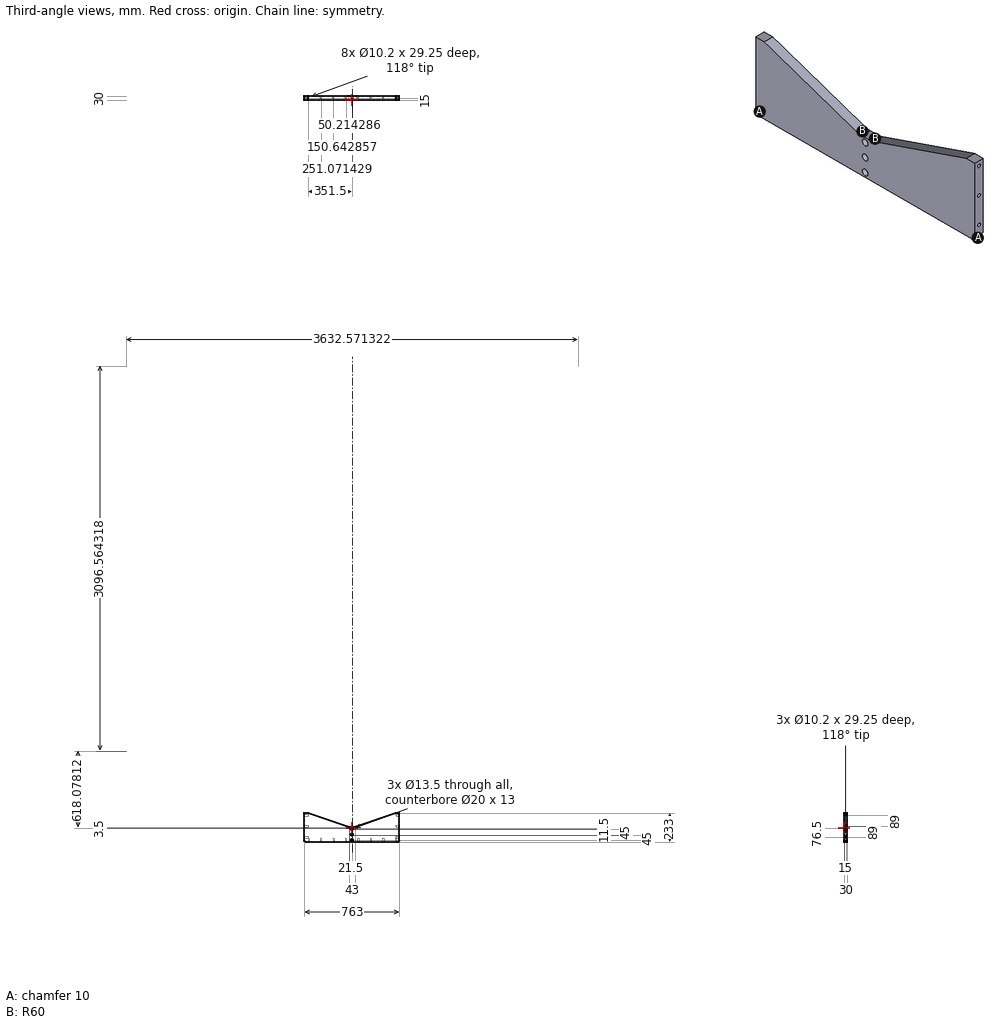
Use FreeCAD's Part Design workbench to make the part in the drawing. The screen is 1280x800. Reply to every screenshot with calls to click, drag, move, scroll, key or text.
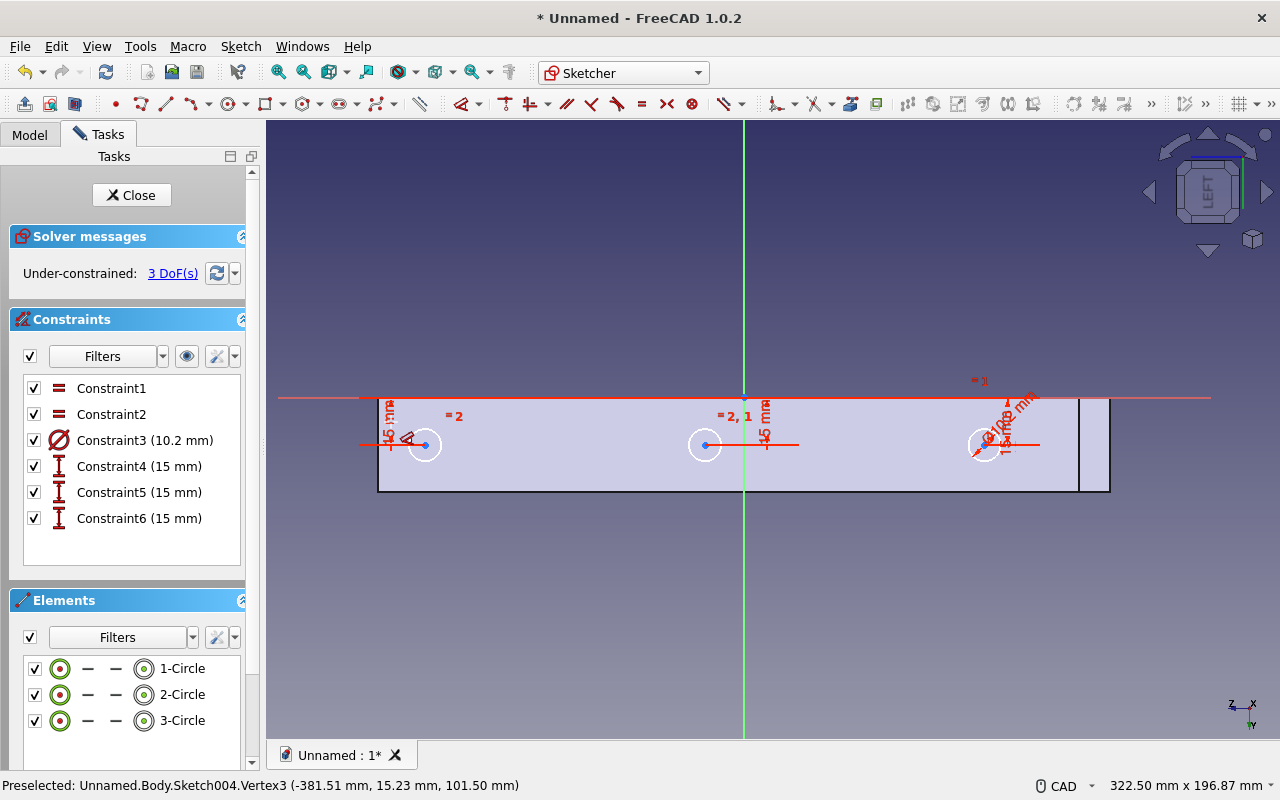
click(985, 445)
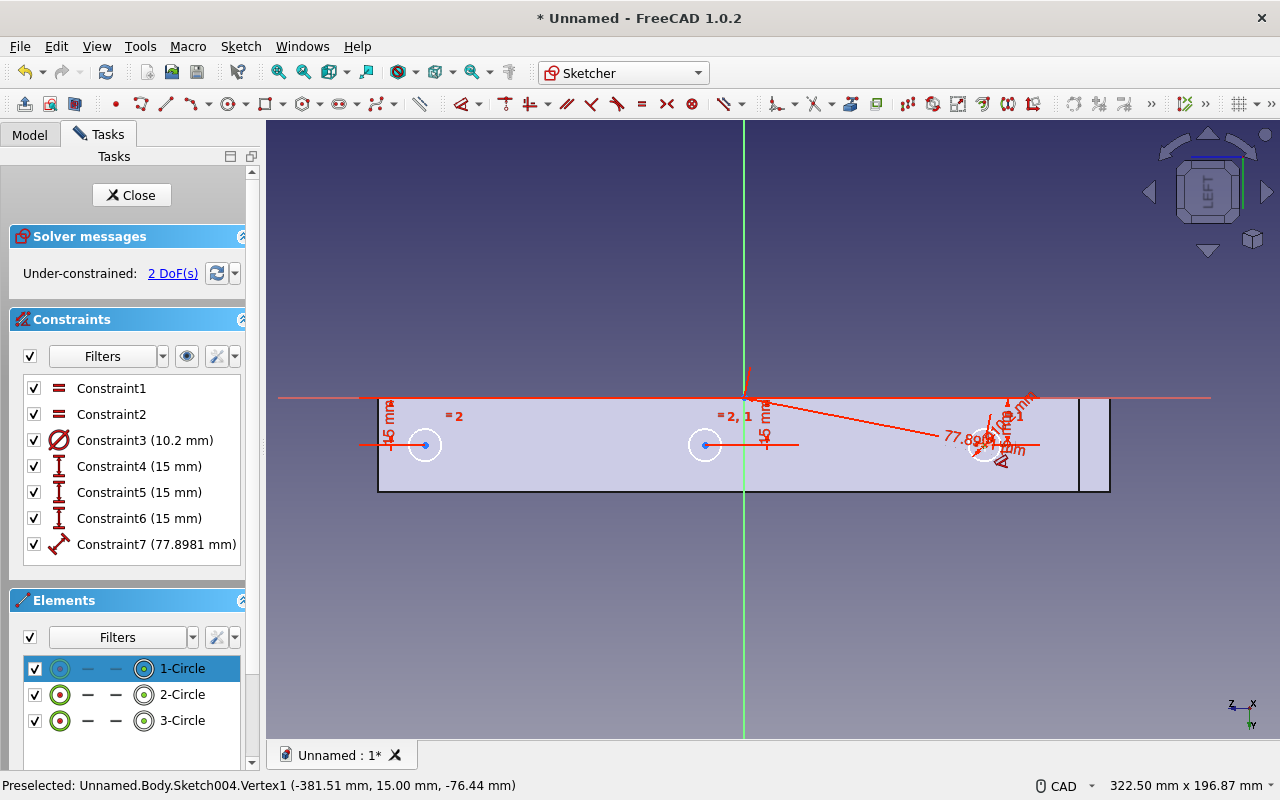
click(705, 445)
click(845, 479)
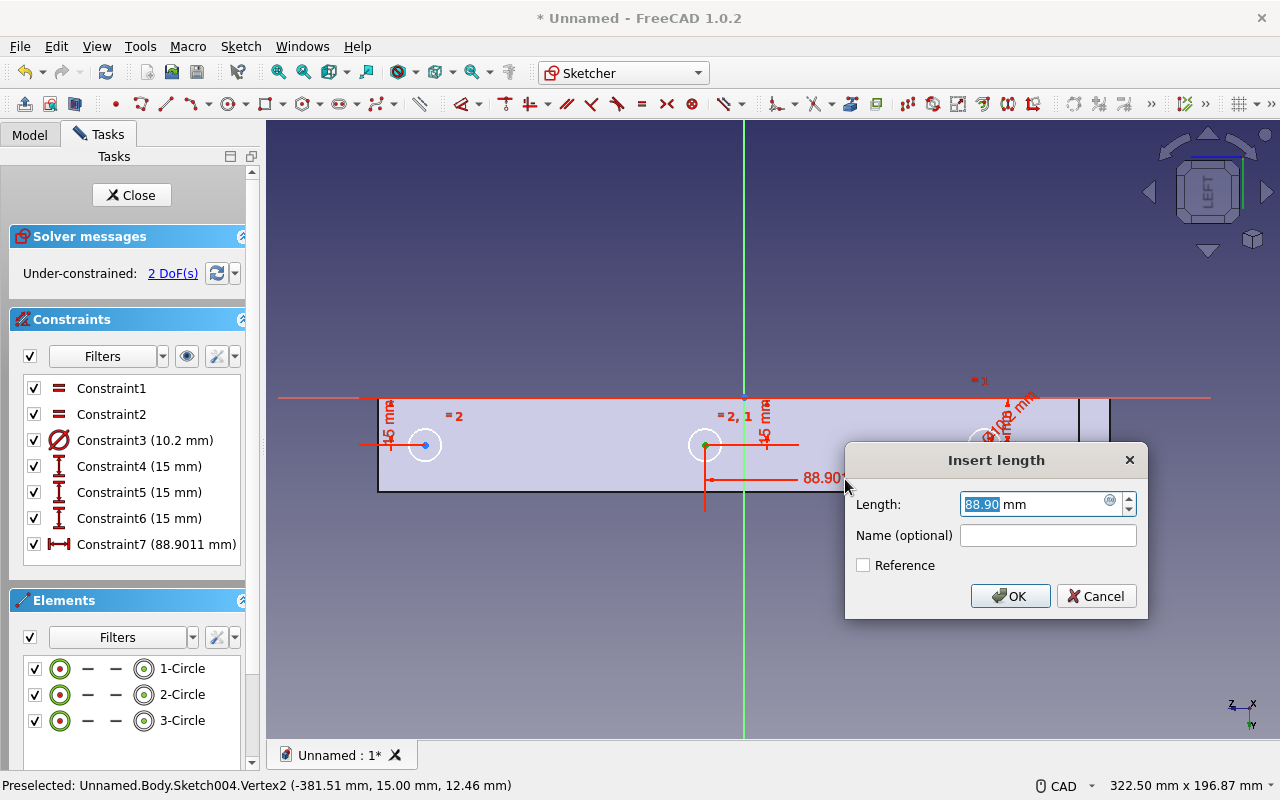
text(89)
key(Return)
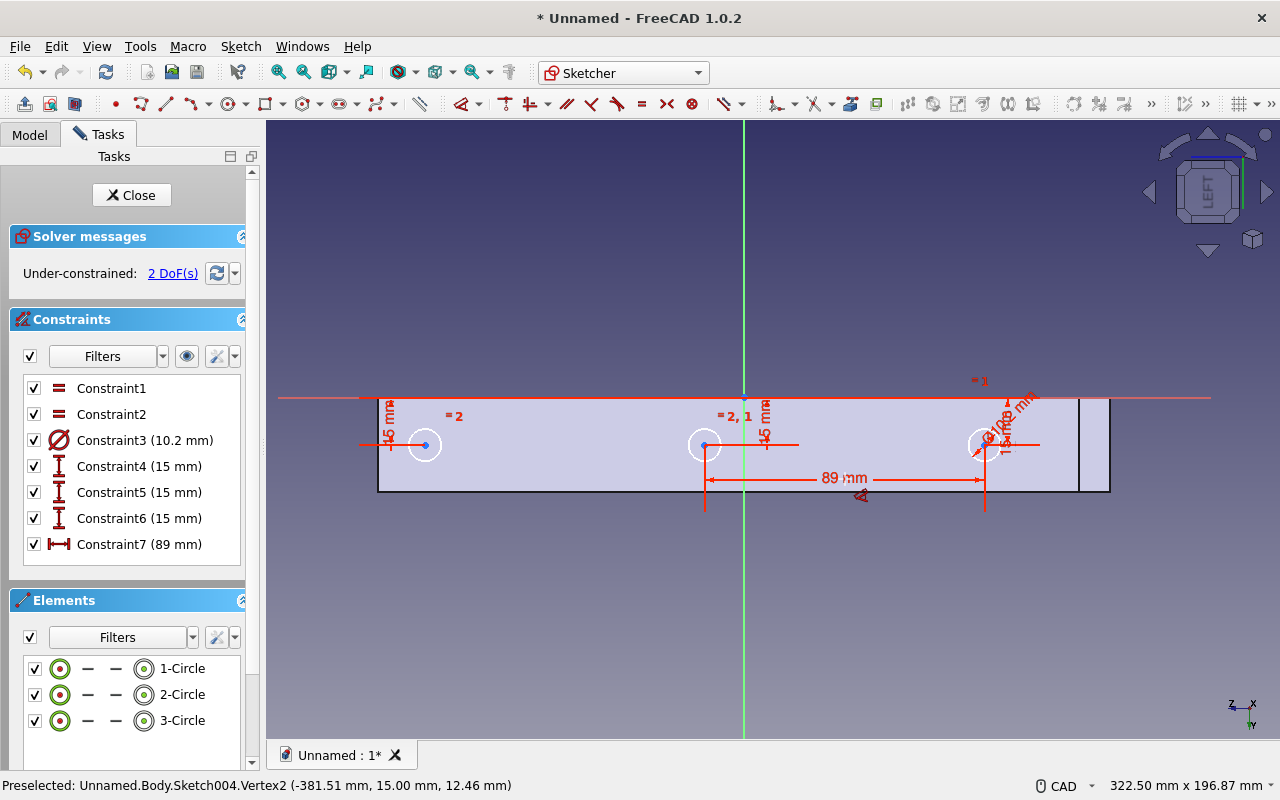
click(705, 445)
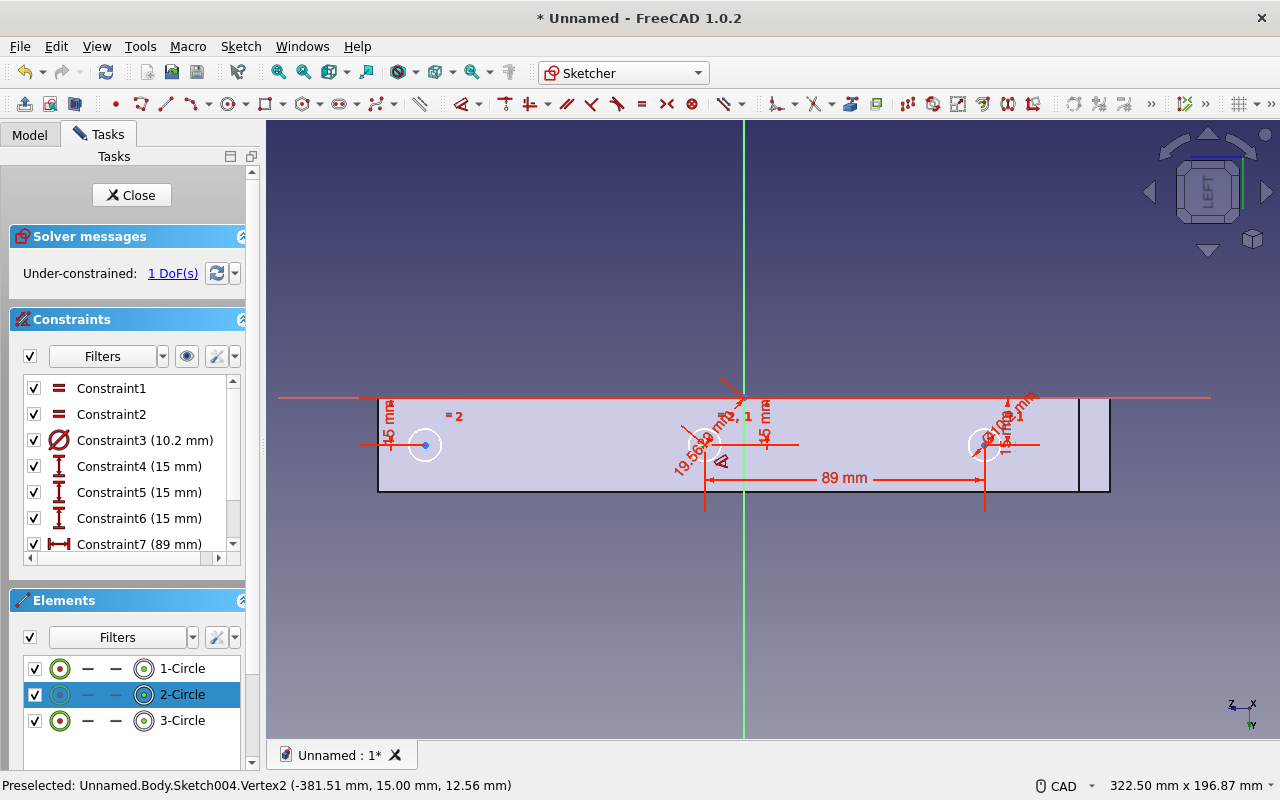
click(425, 445)
click(565, 479)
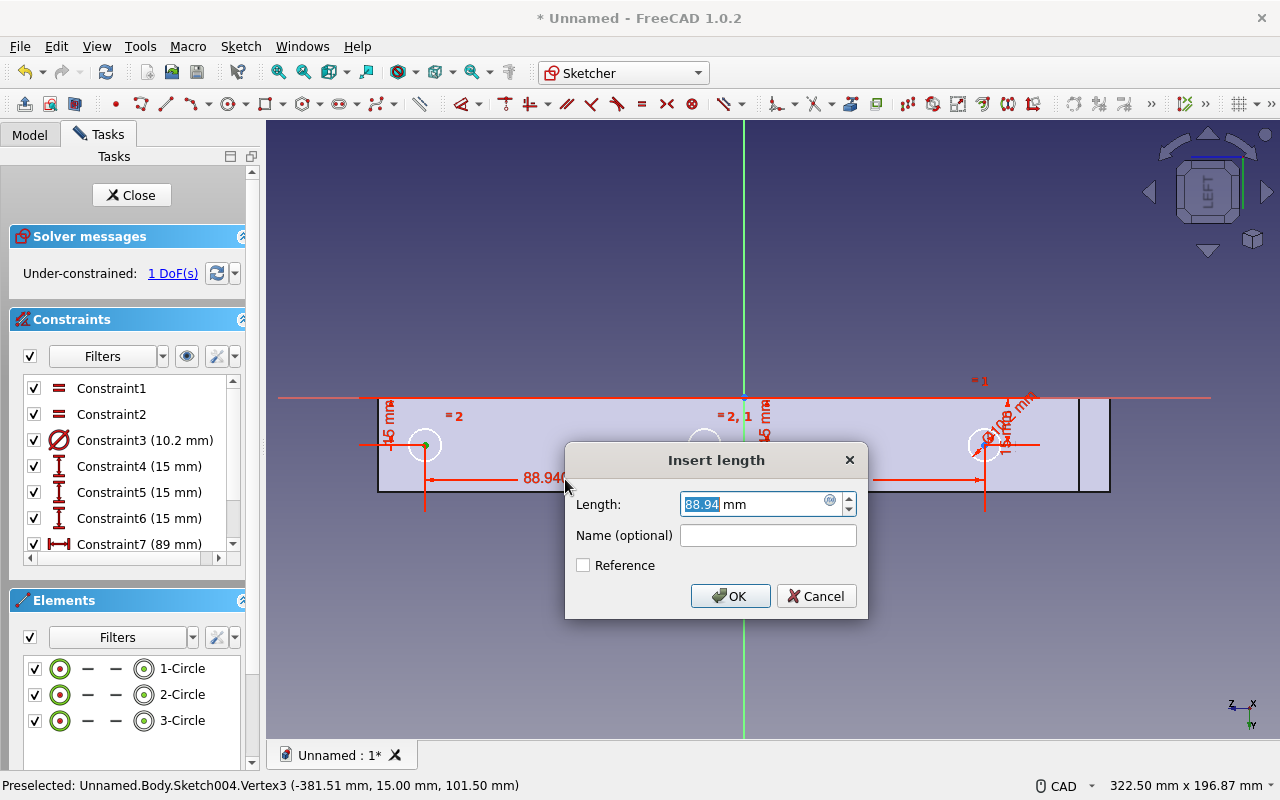
text(89)
key(Return)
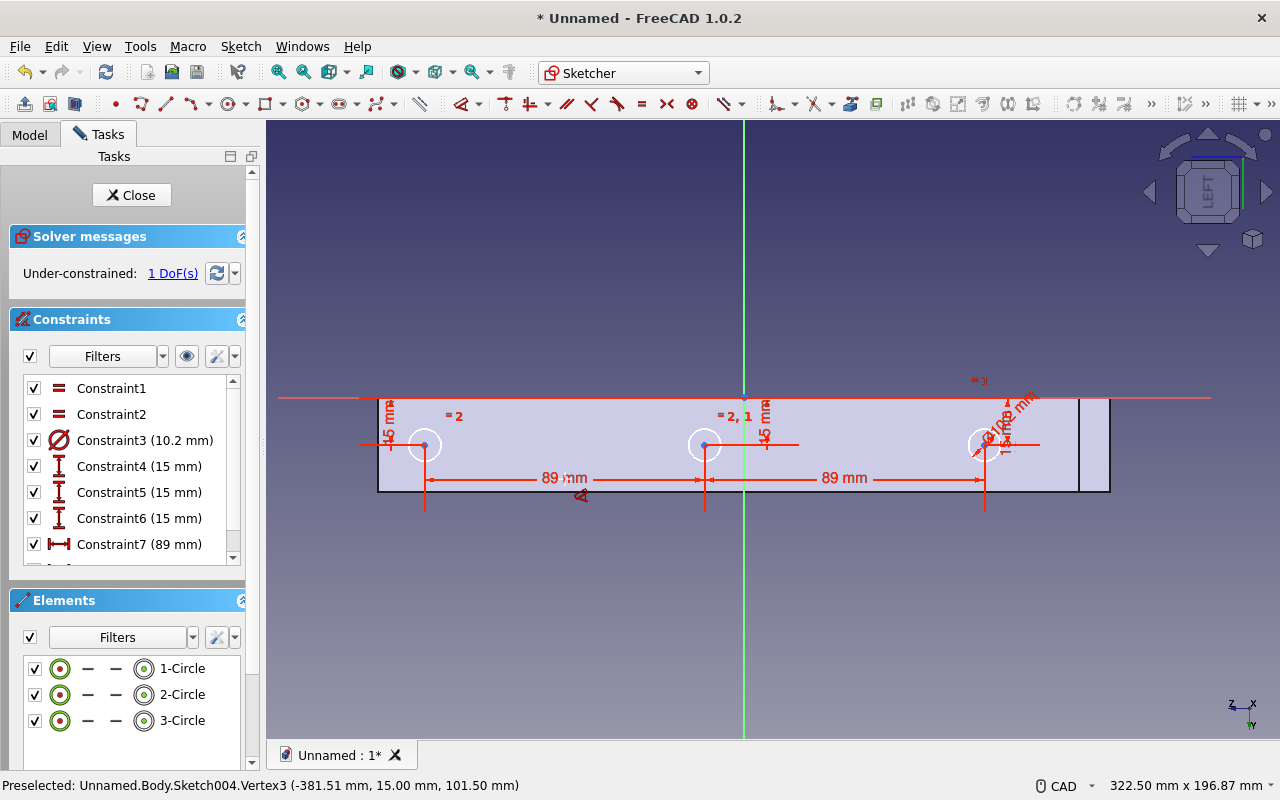
click(985, 445)
click(864, 364)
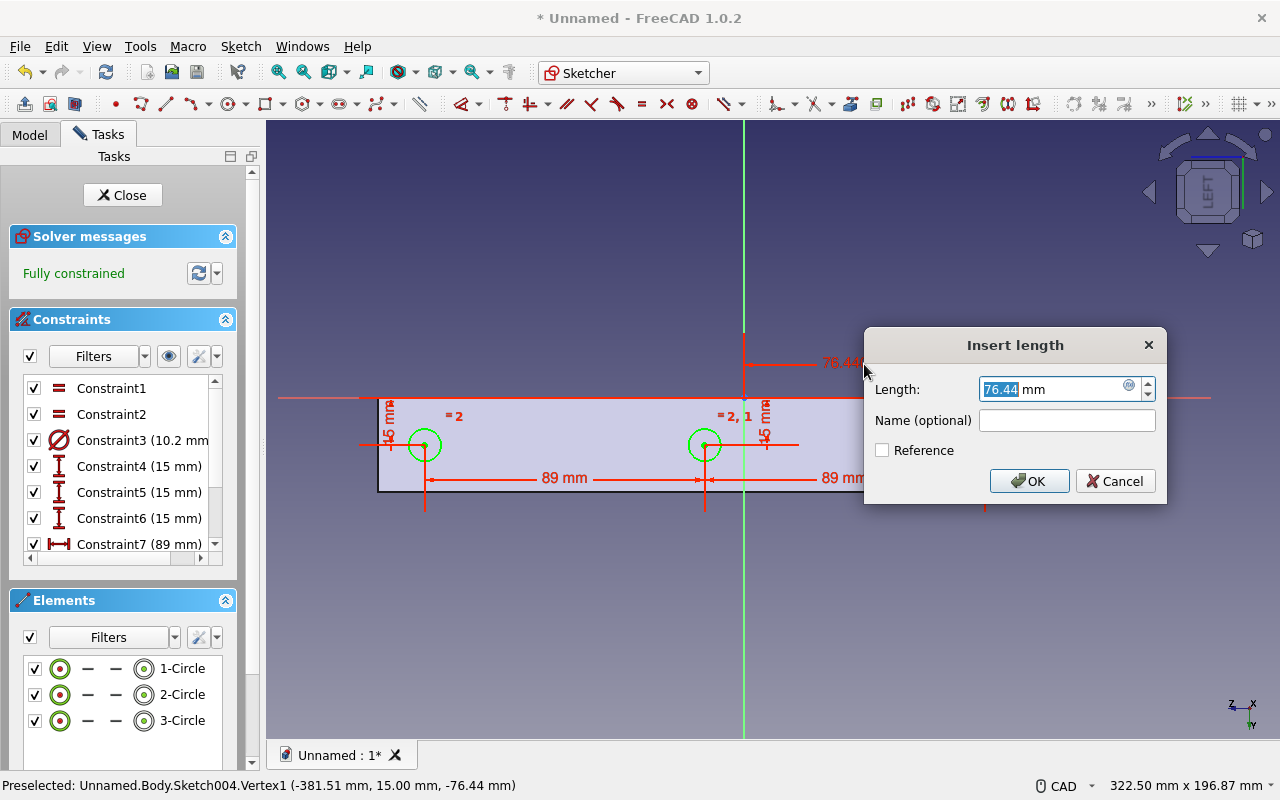
text(76.5)
key(Return)
key(Escape)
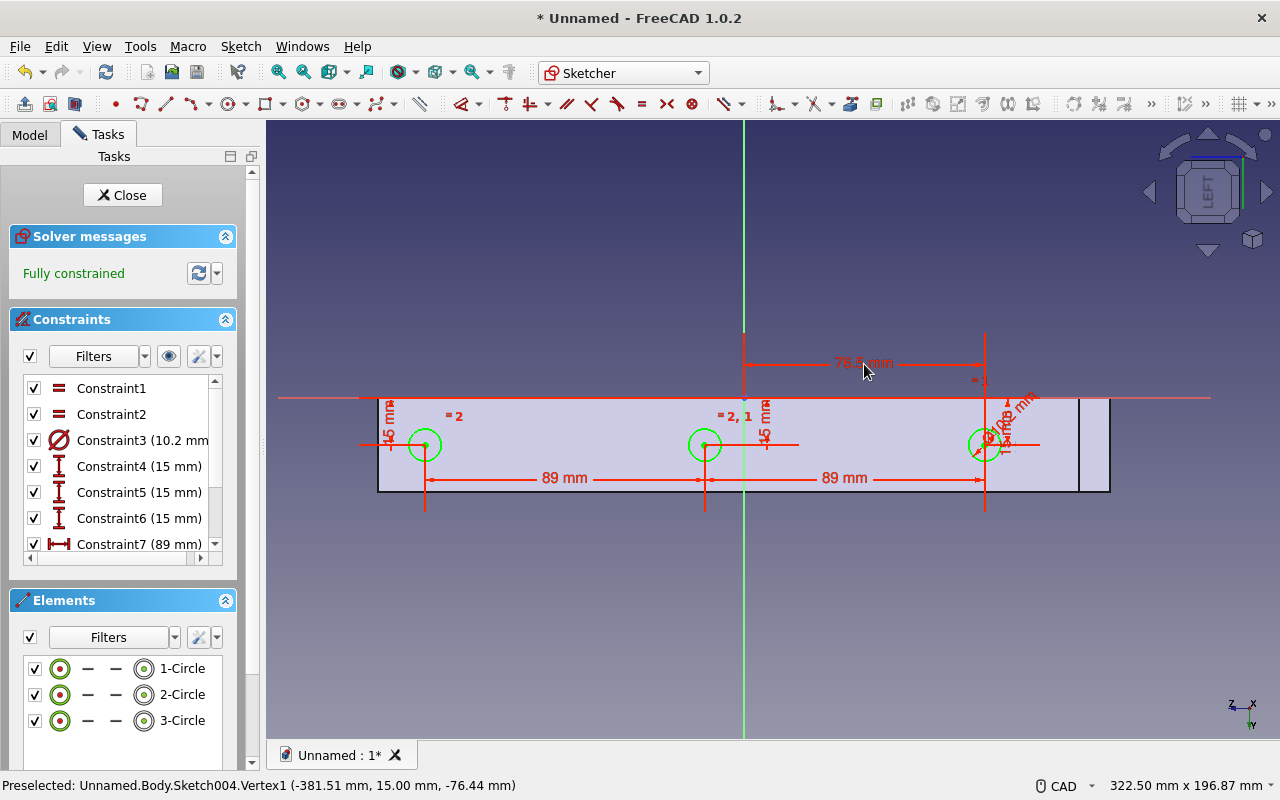
click(123, 195)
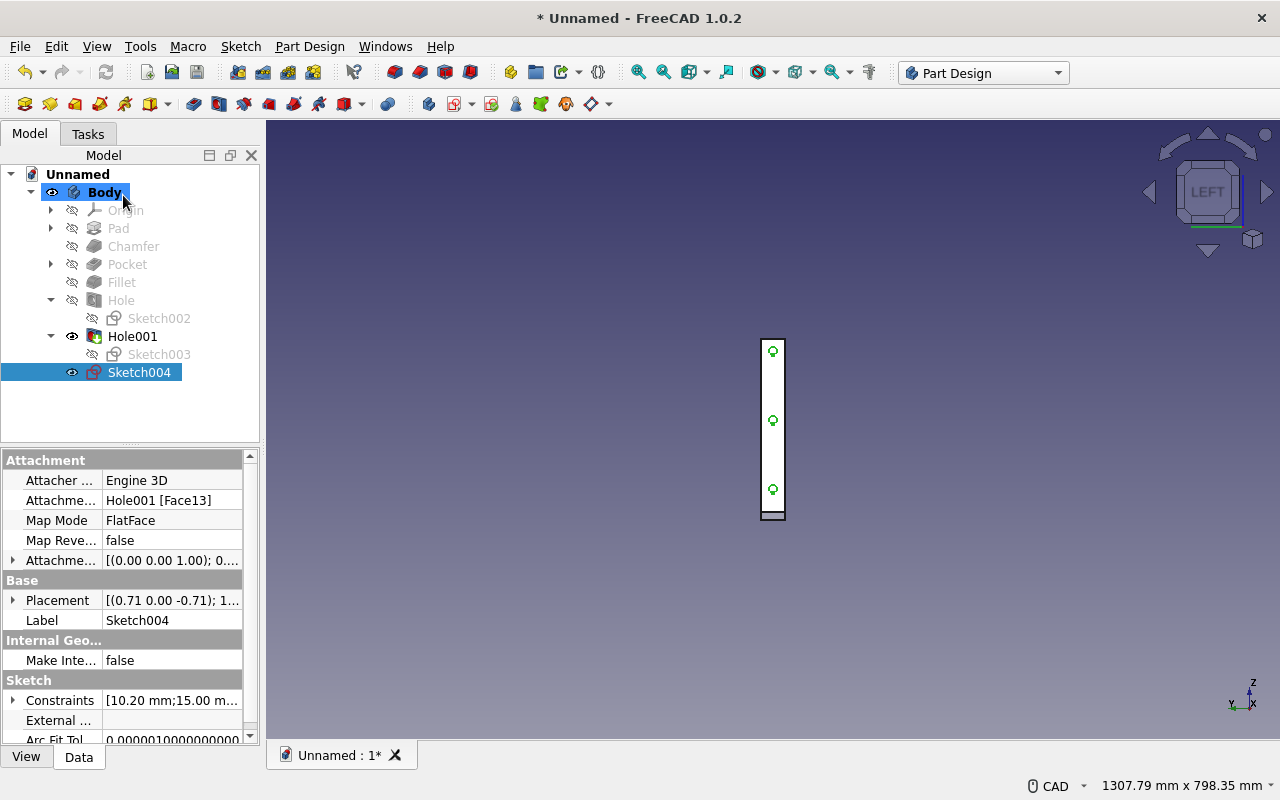
click(219, 104)